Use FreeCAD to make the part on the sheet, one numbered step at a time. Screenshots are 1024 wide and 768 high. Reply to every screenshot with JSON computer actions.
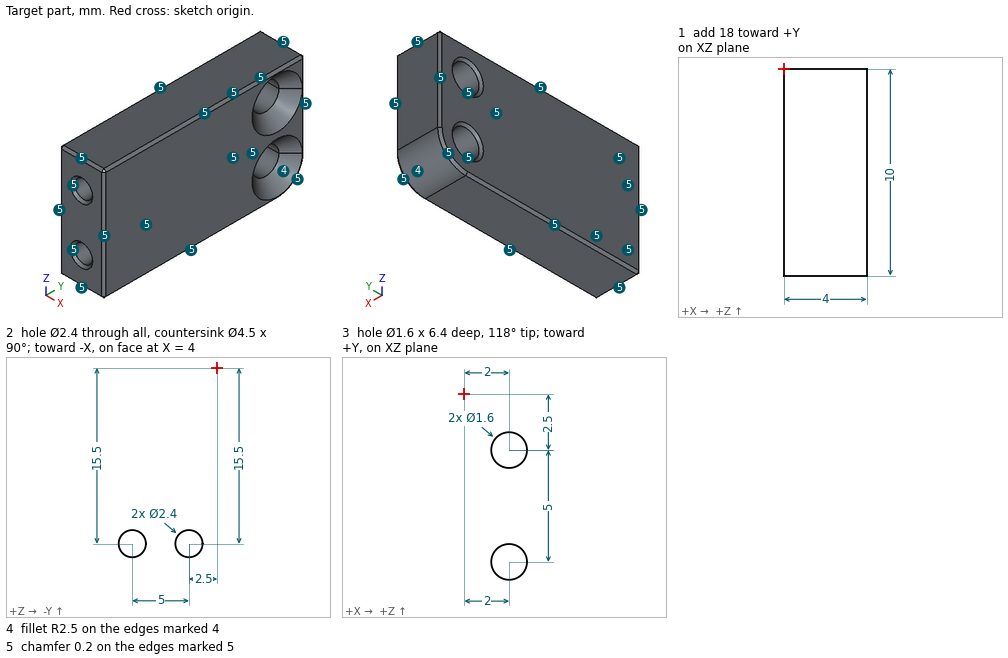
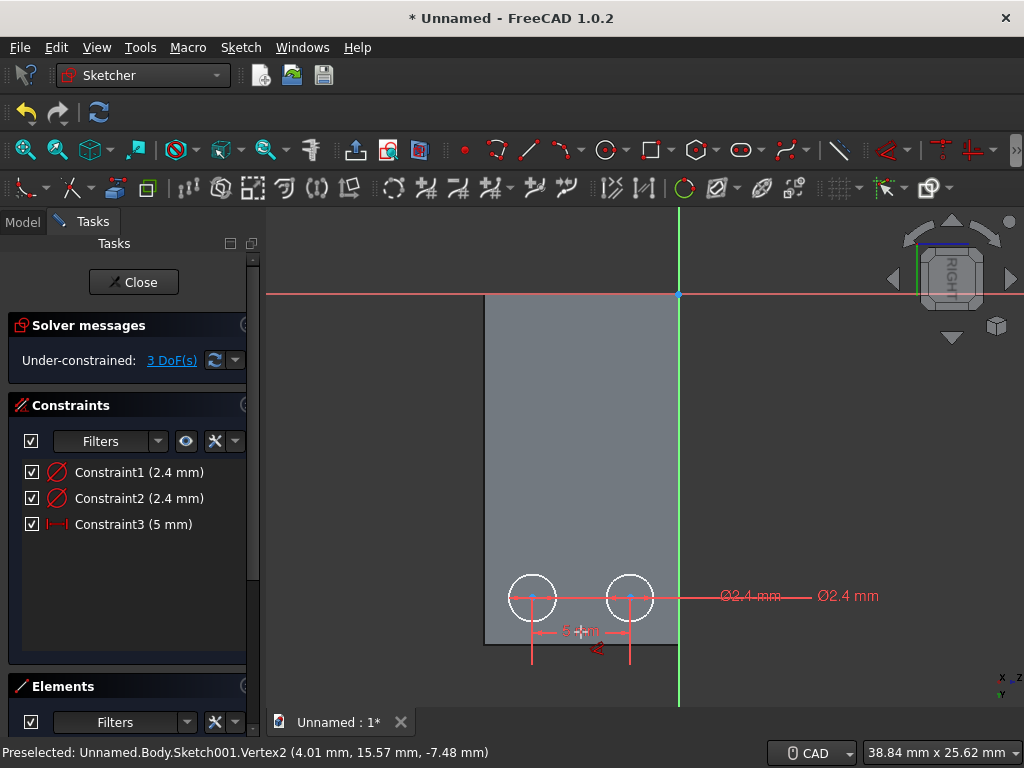
{"action": "left_click", "coordinate": [630, 598]}
{"action": "left_click", "coordinate": [654, 260]}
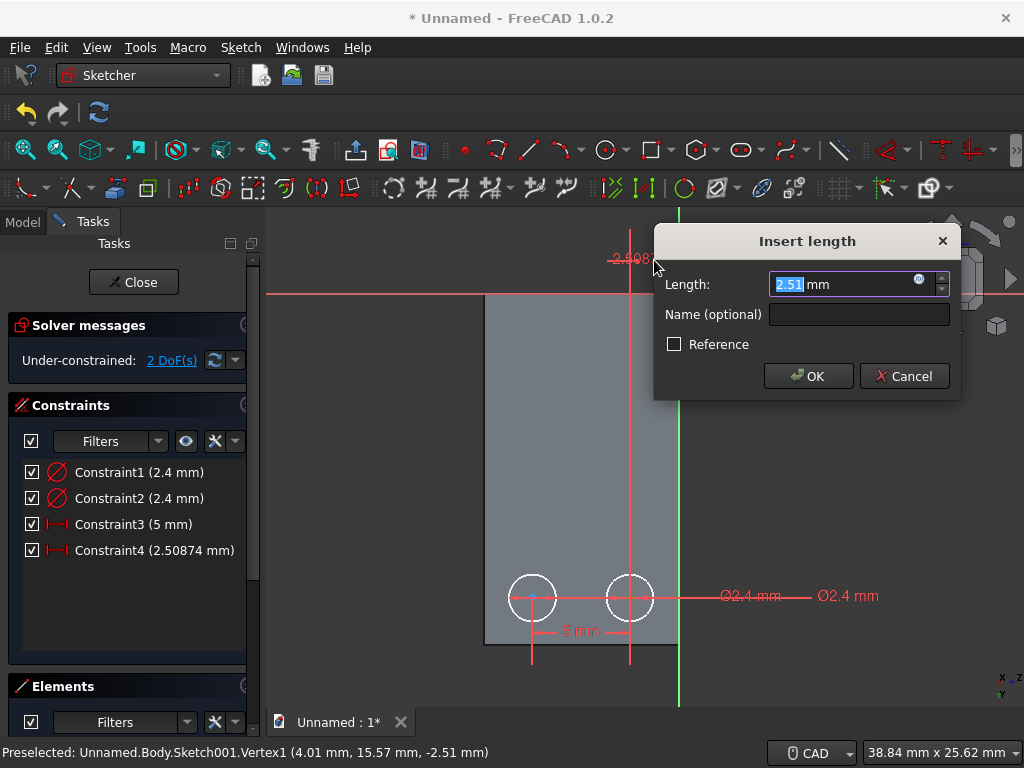
{"action": "type", "text": "2.5"}
{"action": "key", "text": "Return"}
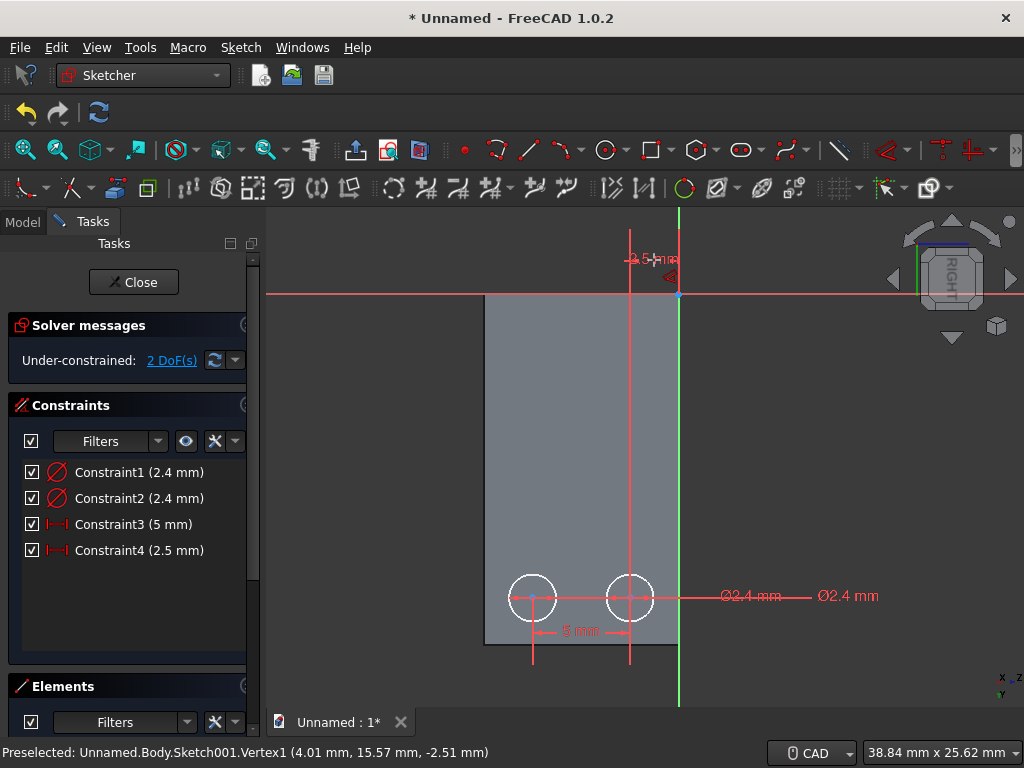
{"action": "left_click", "coordinate": [630, 598]}
{"action": "left_click", "coordinate": [713, 446]}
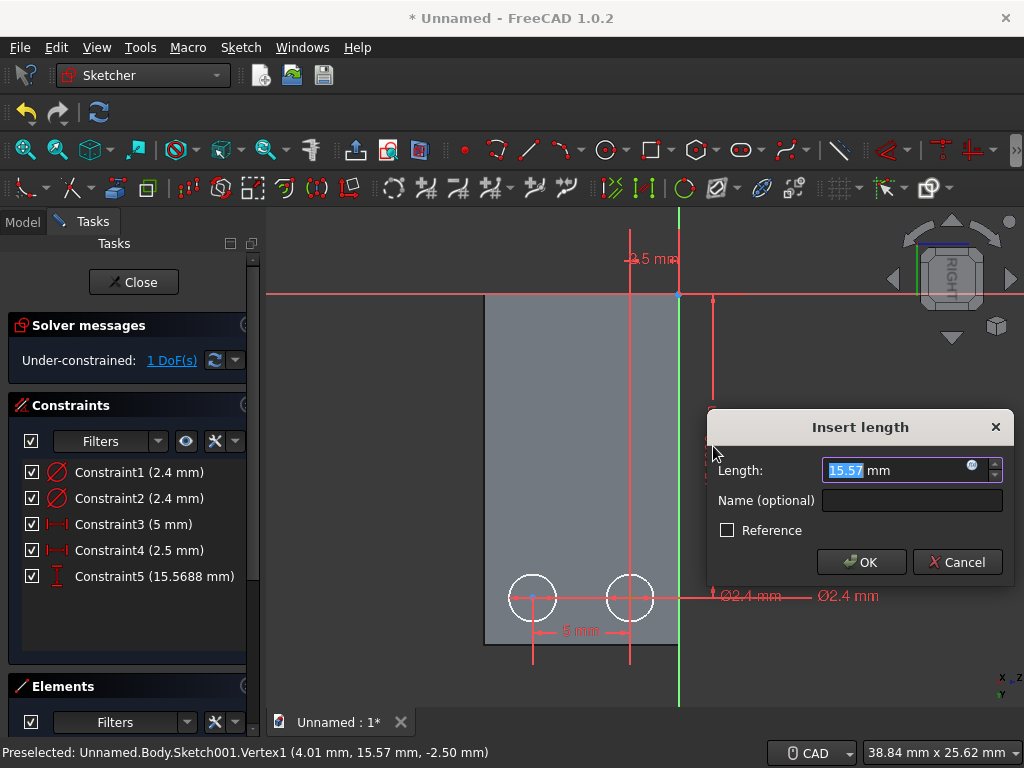
{"action": "type", "text": "15.5"}
{"action": "key", "text": "Return"}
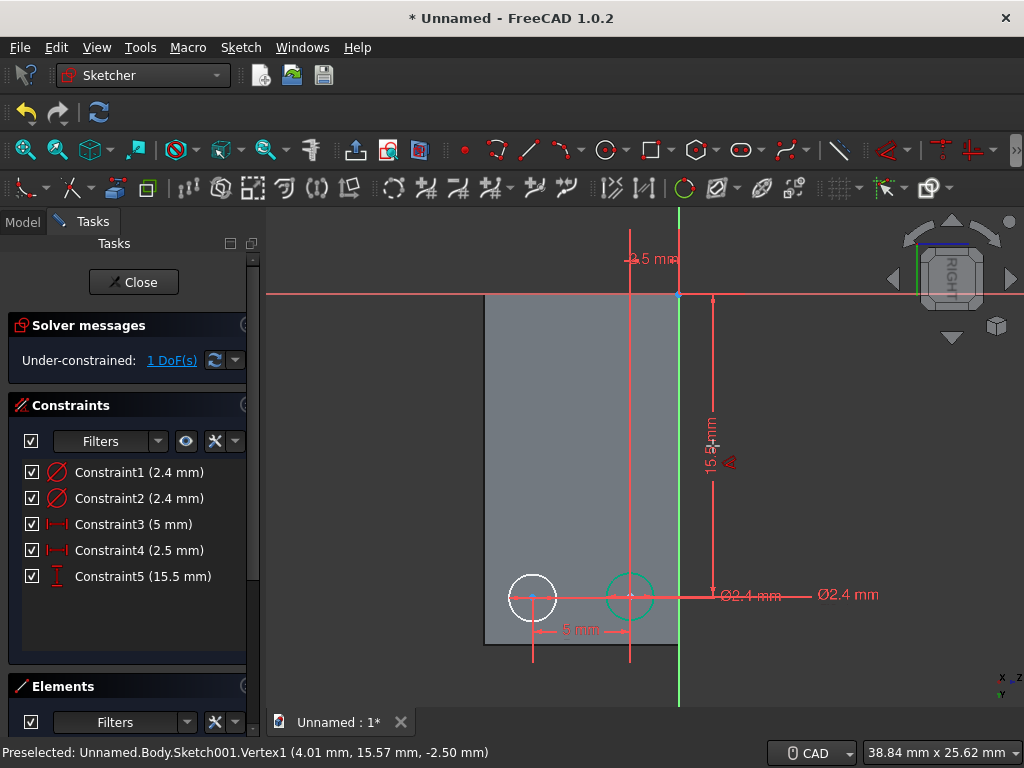
{"action": "left_click", "coordinate": [533, 598]}
{"action": "left_click", "coordinate": [713, 376]}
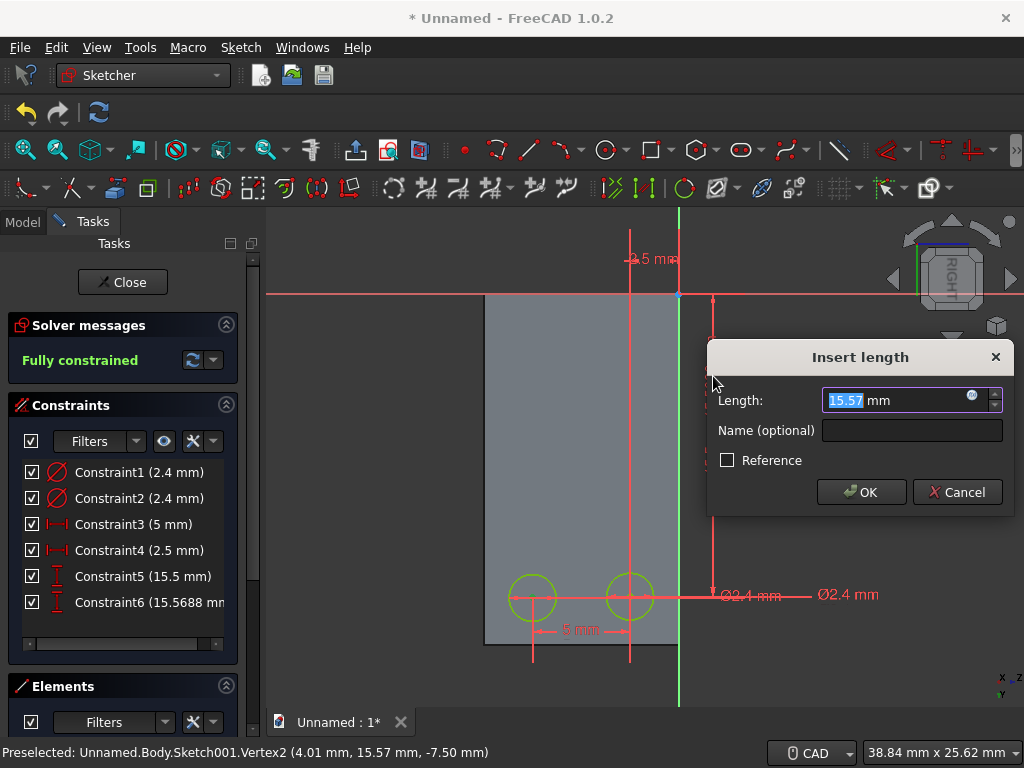
{"action": "type", "text": "15.5"}
{"action": "key", "text": "Return"}
{"action": "key", "text": "Escape"}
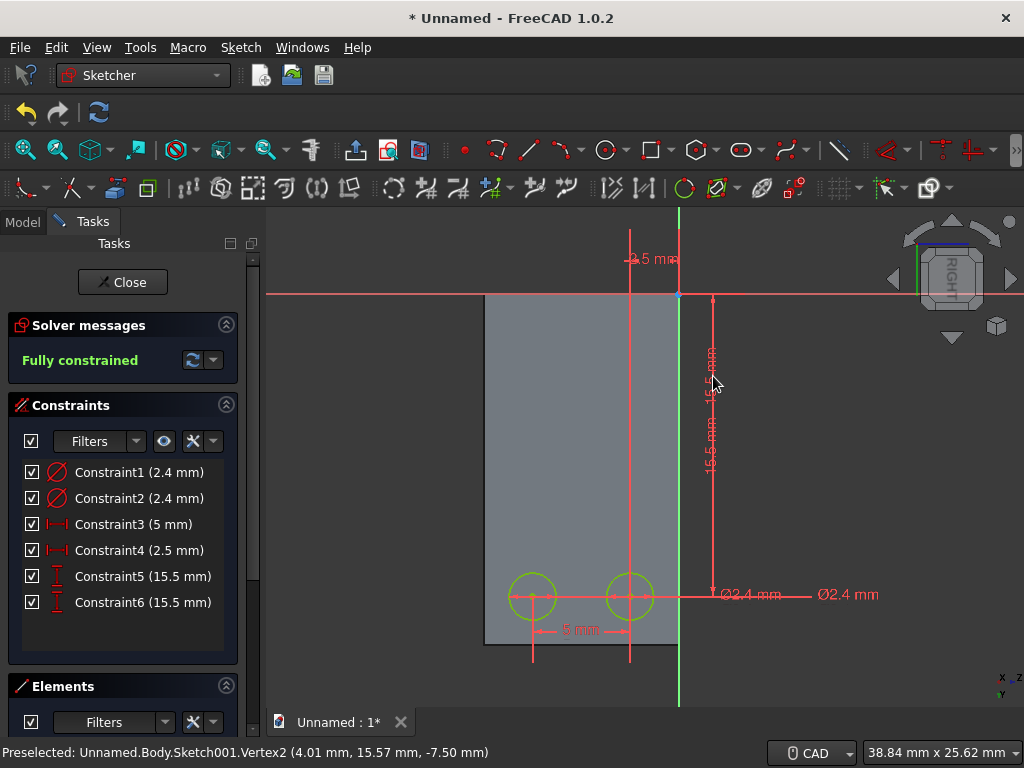
{"action": "left_click", "coordinate": [123, 282]}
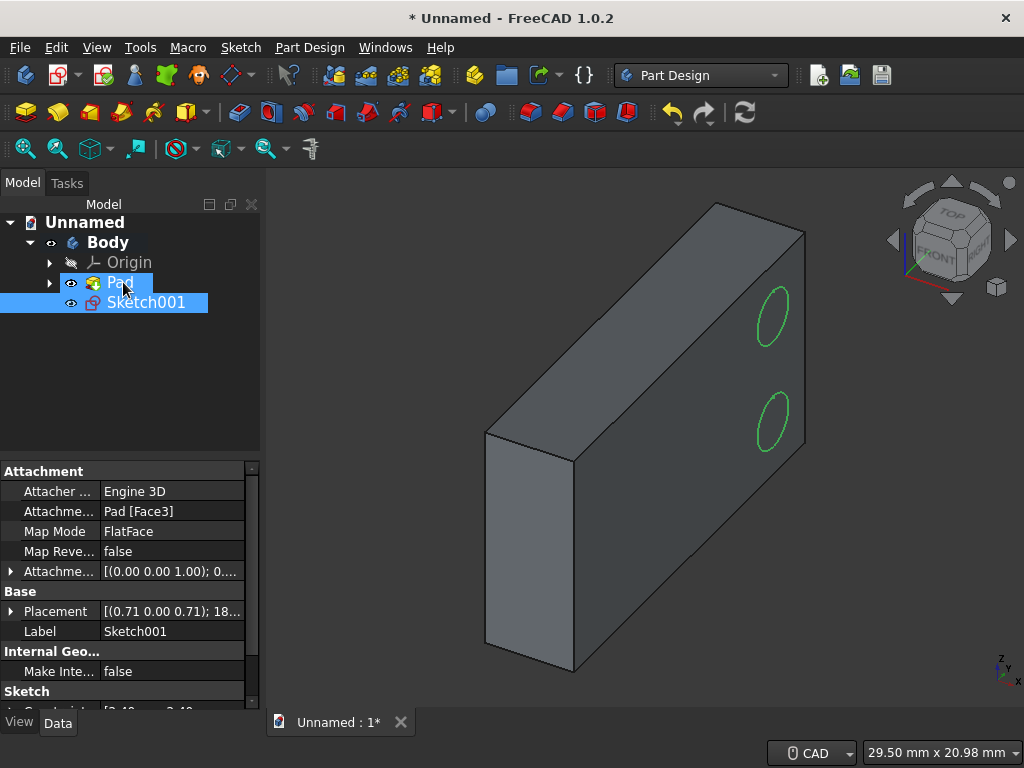
{"action": "left_click", "coordinate": [272, 112]}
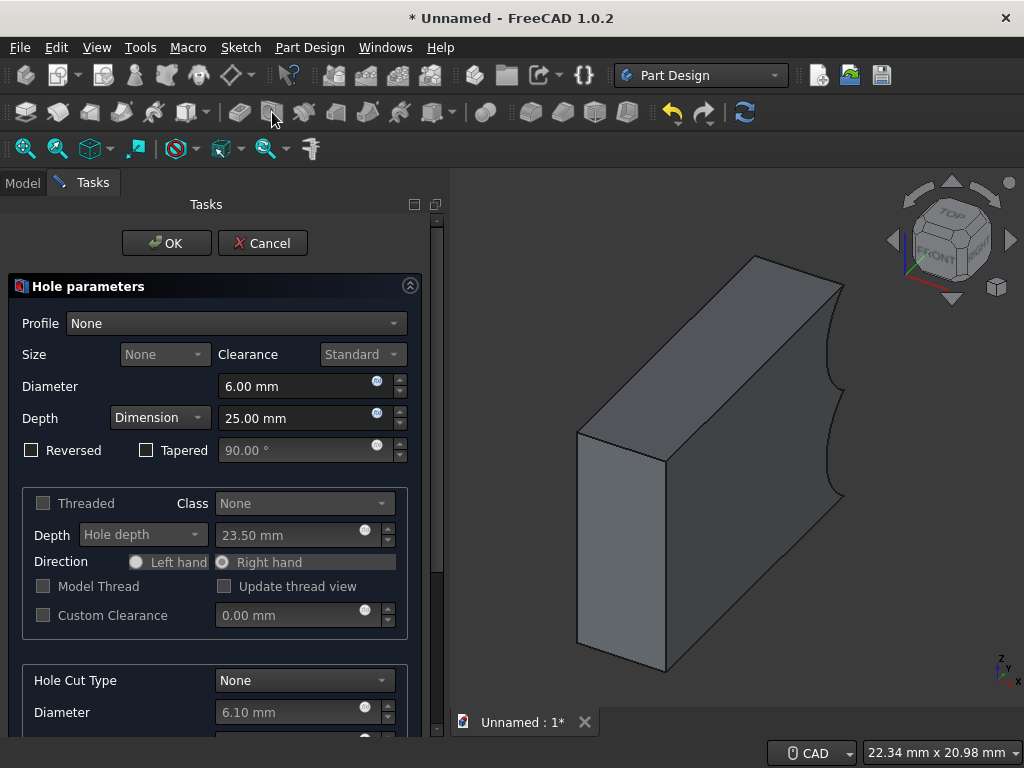
{"action": "triple_click", "coordinate": [305, 386]}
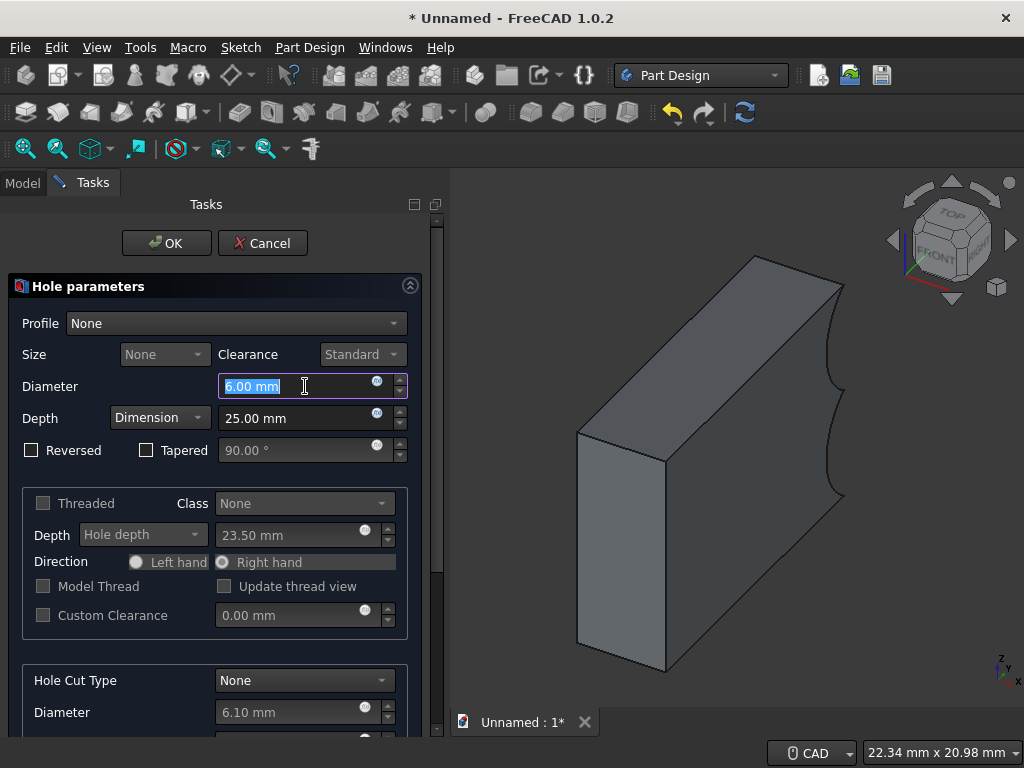
{"action": "type", "text": "2.4"}
{"action": "key", "text": "Tab"}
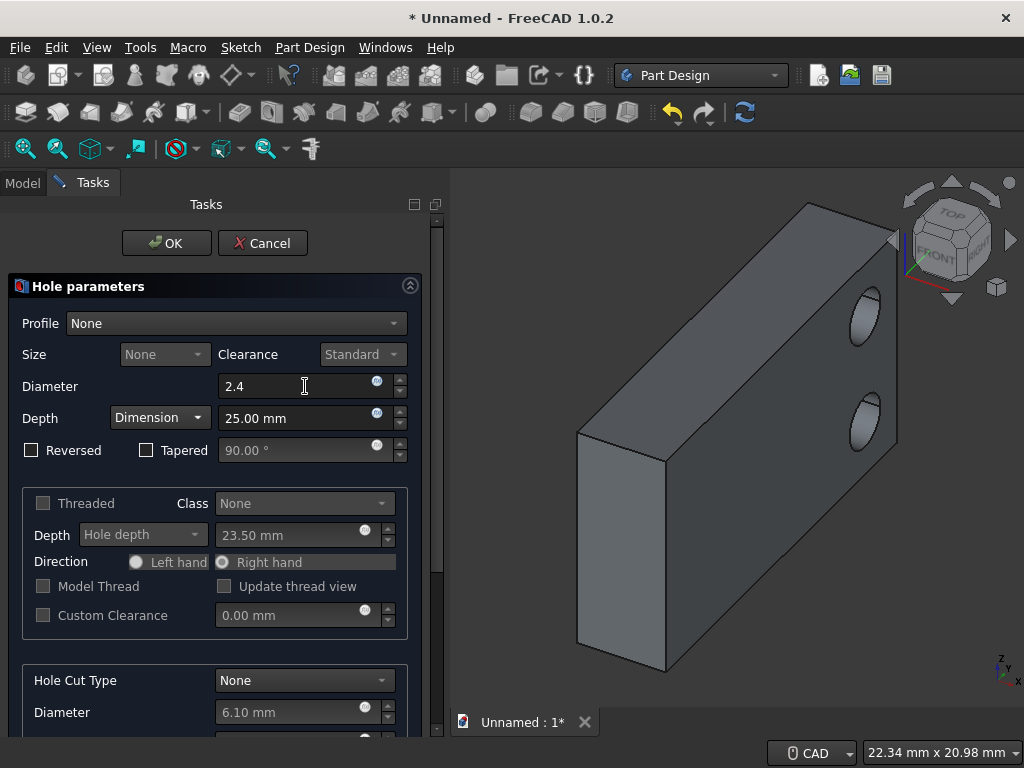
{"action": "left_click", "coordinate": [161, 418]}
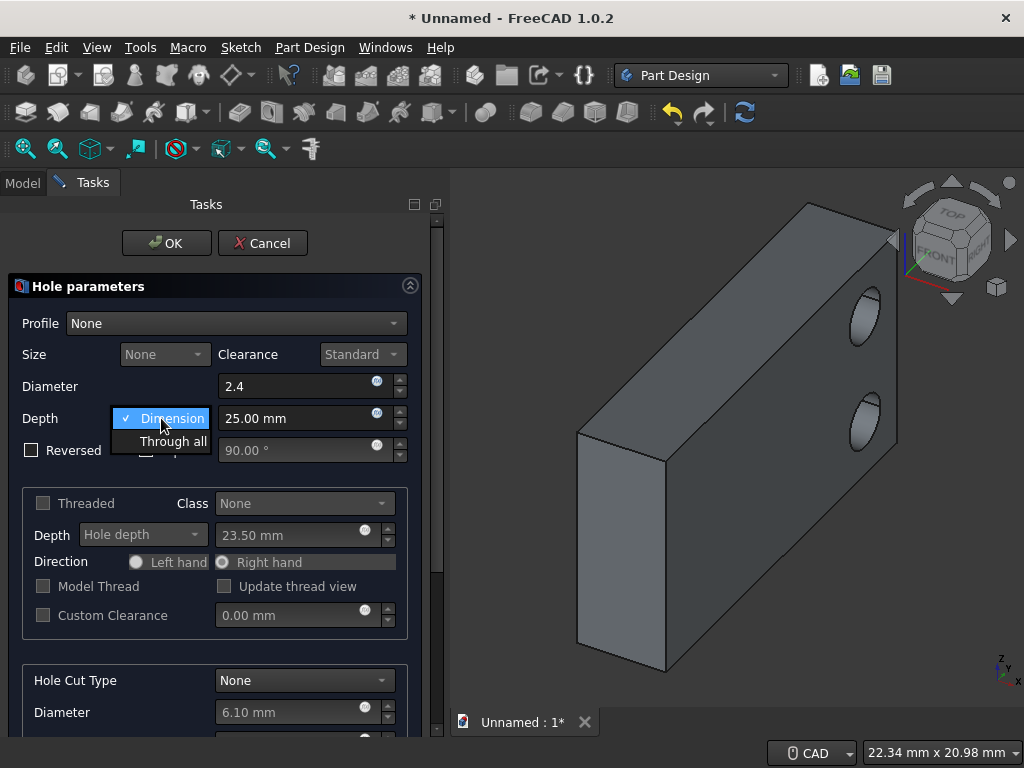
{"action": "left_click", "coordinate": [160, 442]}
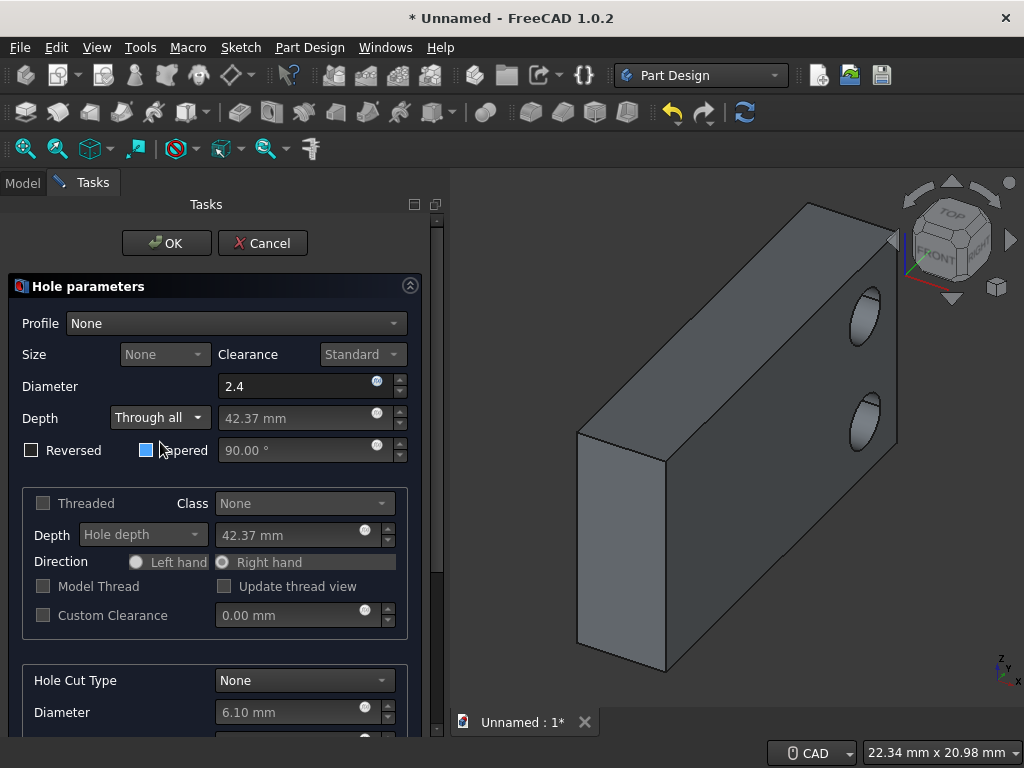
{"action": "left_click", "coordinate": [306, 680]}